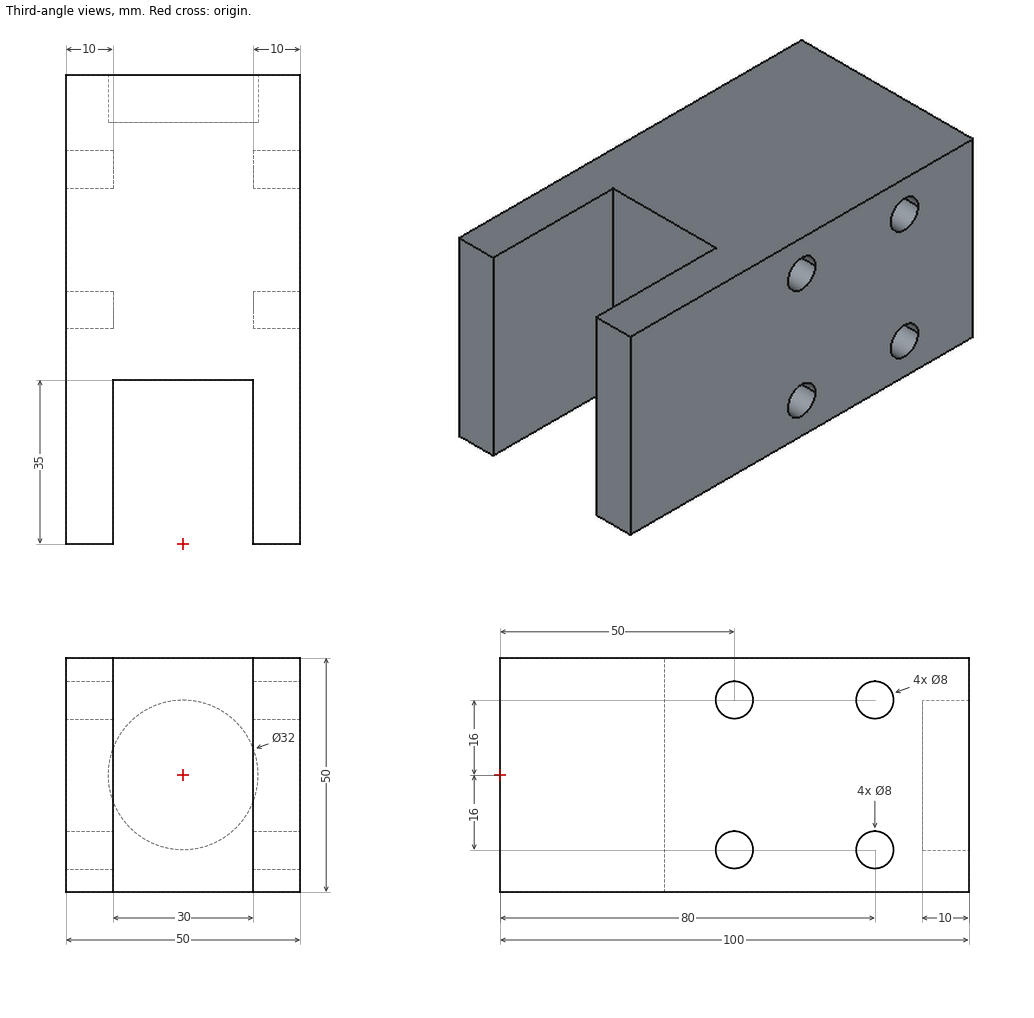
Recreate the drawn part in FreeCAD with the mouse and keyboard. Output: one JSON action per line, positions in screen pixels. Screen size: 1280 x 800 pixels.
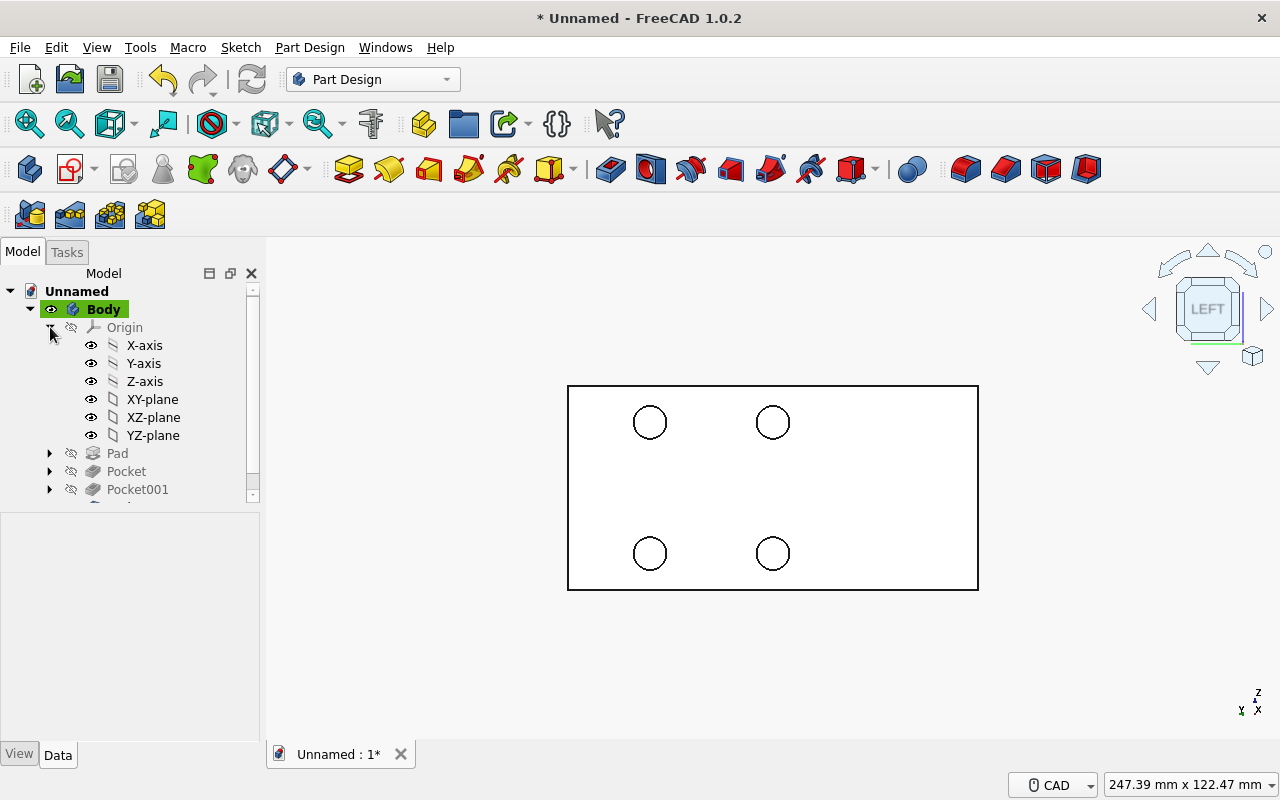
{"action": "left_click", "coordinate": [136, 435]}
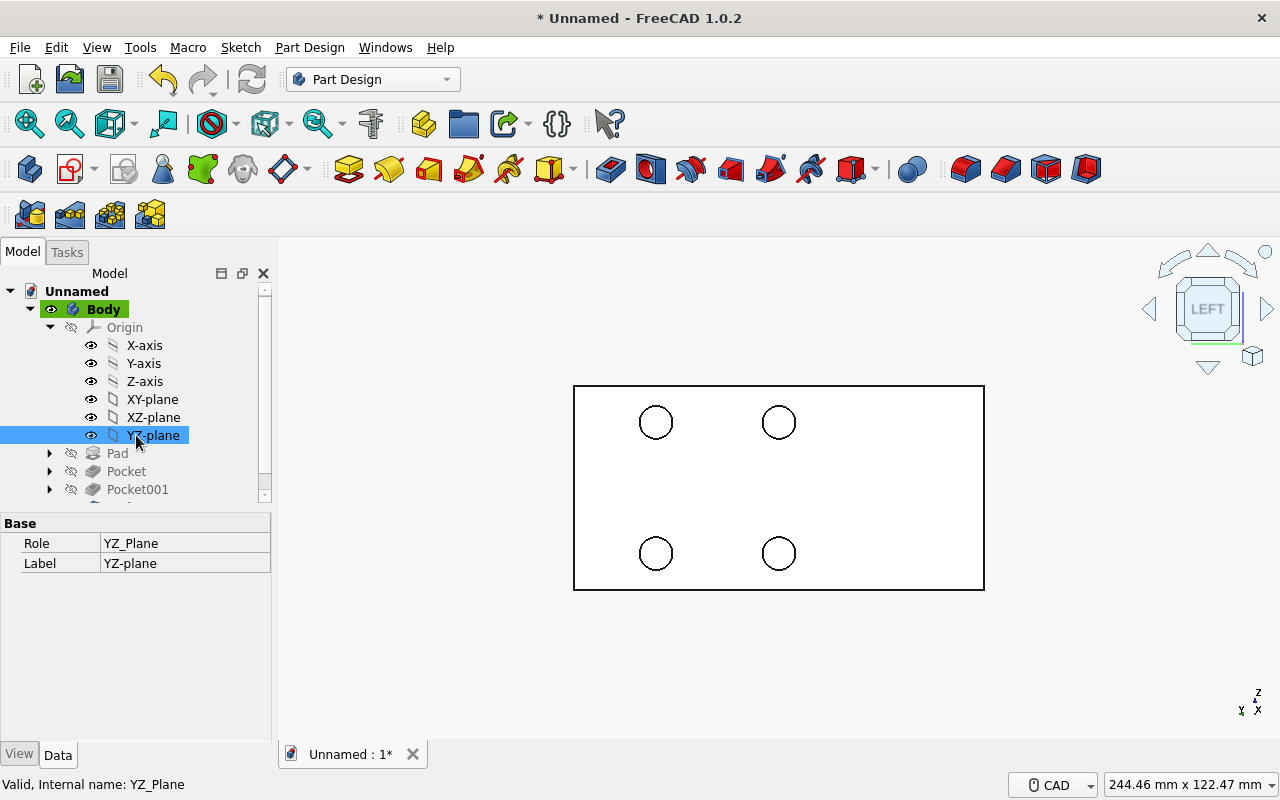
{"action": "left_click", "coordinate": [284, 170]}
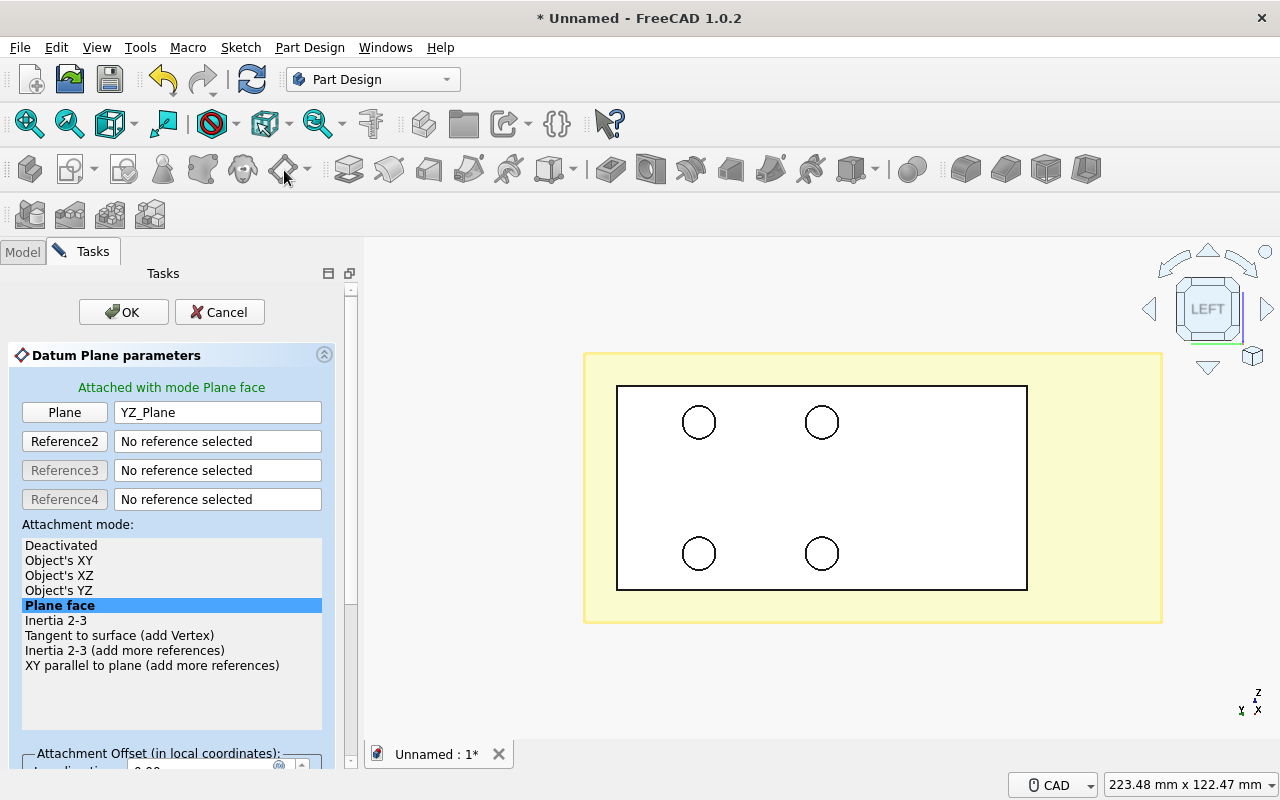
{"action": "scroll", "coordinate": [351, 526], "scroll_direction": "down", "scroll_amount": 3}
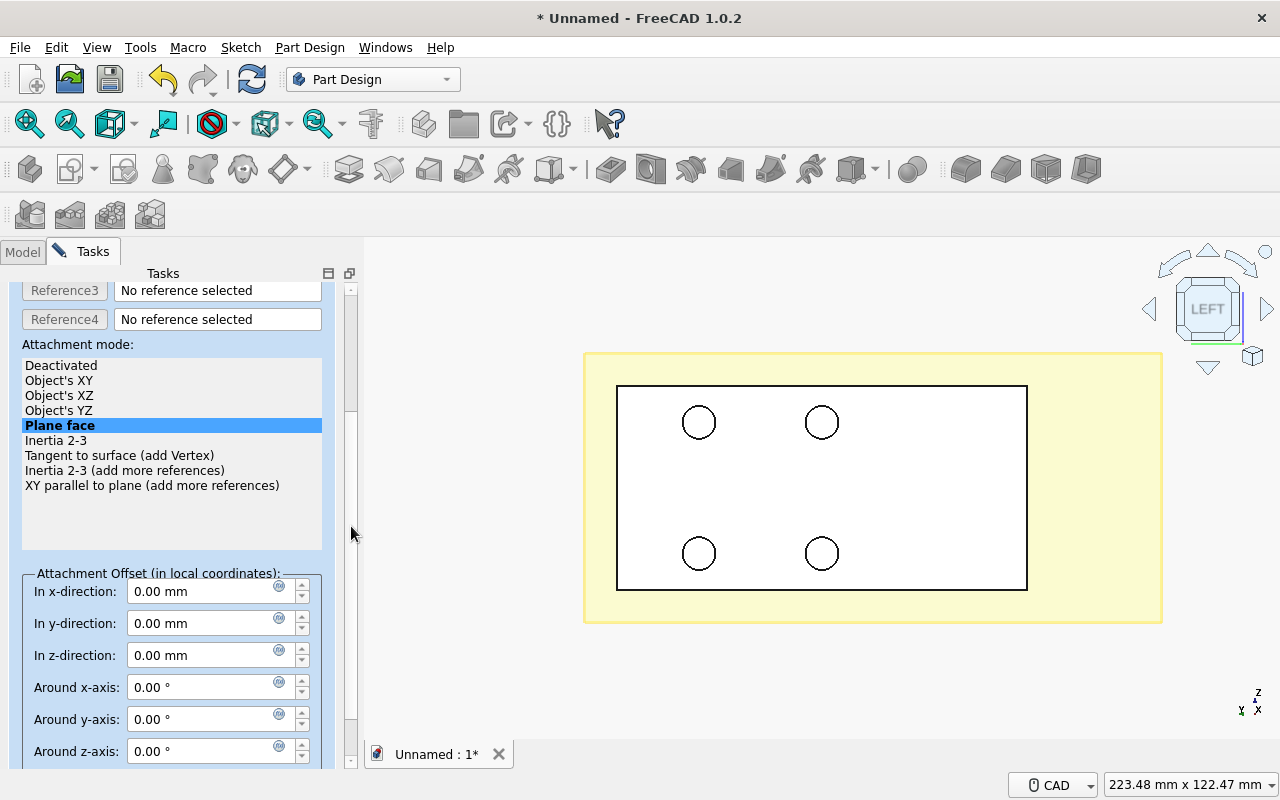
{"action": "triple_click", "coordinate": [210, 655]}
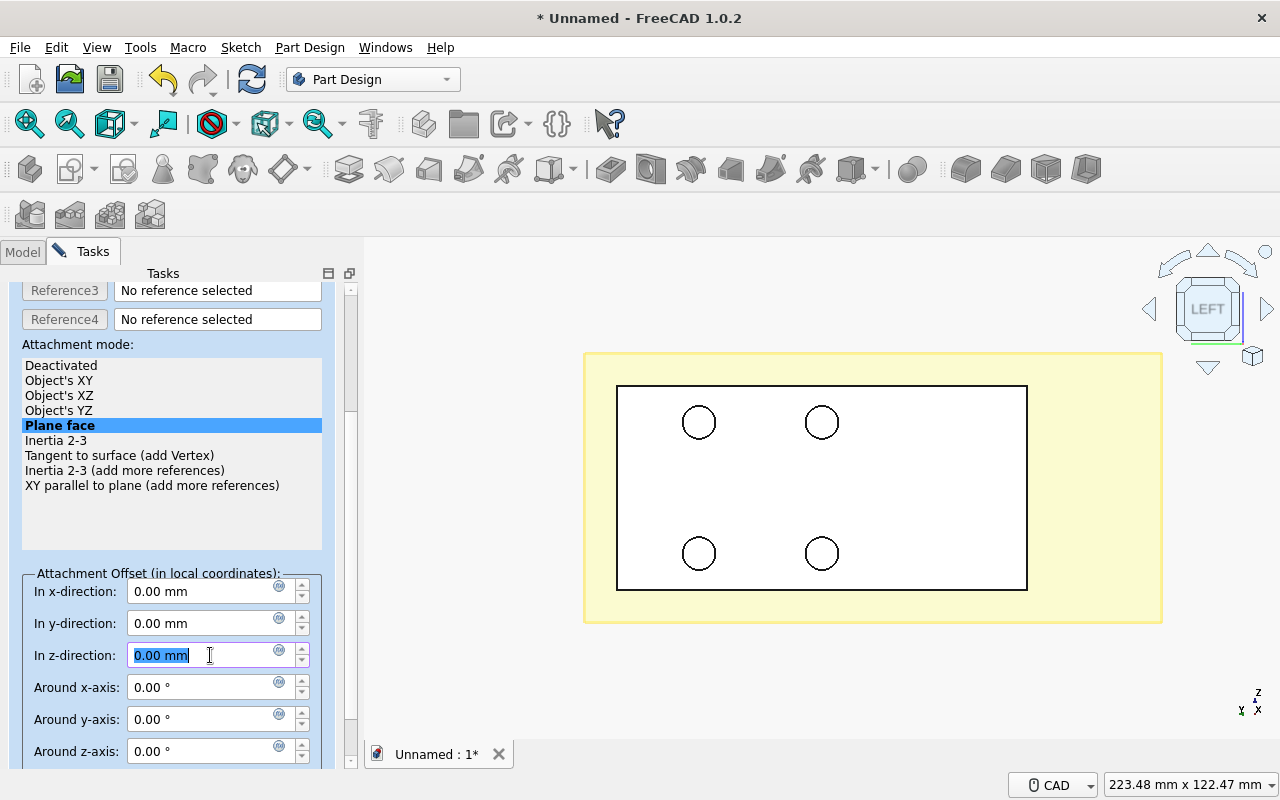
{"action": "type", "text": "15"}
{"action": "key", "text": "Tab"}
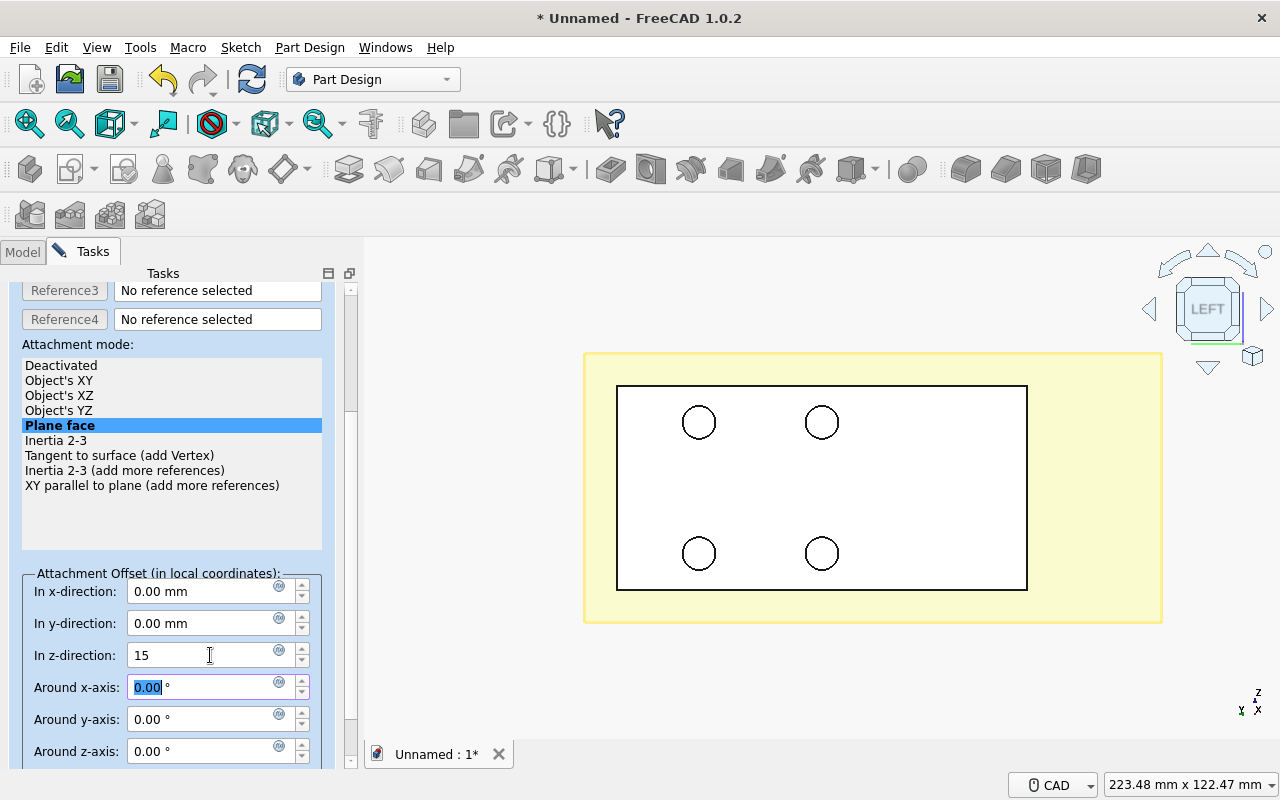
{"action": "scroll", "coordinate": [351, 526], "scroll_direction": "up", "scroll_amount": 4}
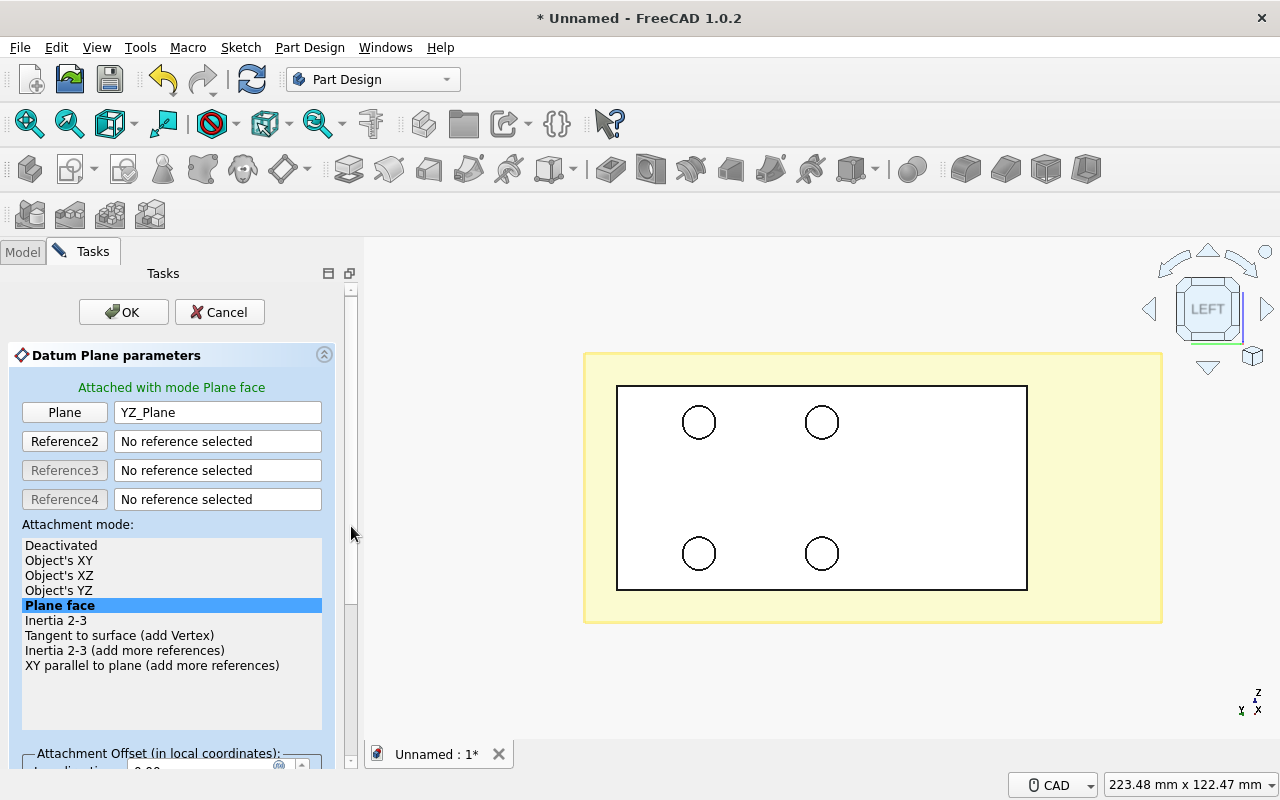
{"action": "left_click", "coordinate": [124, 312]}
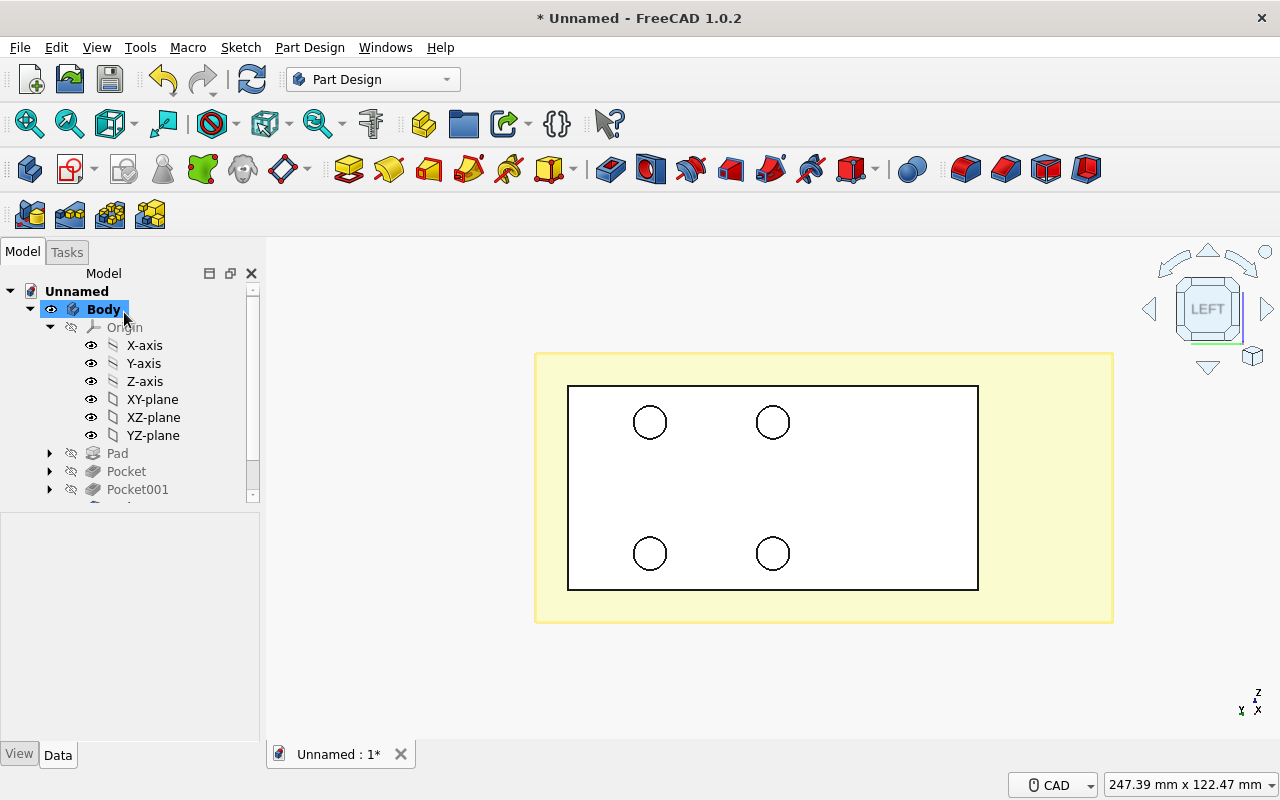
{"action": "scroll", "coordinate": [100, 395], "scroll_direction": "down", "scroll_amount": 3}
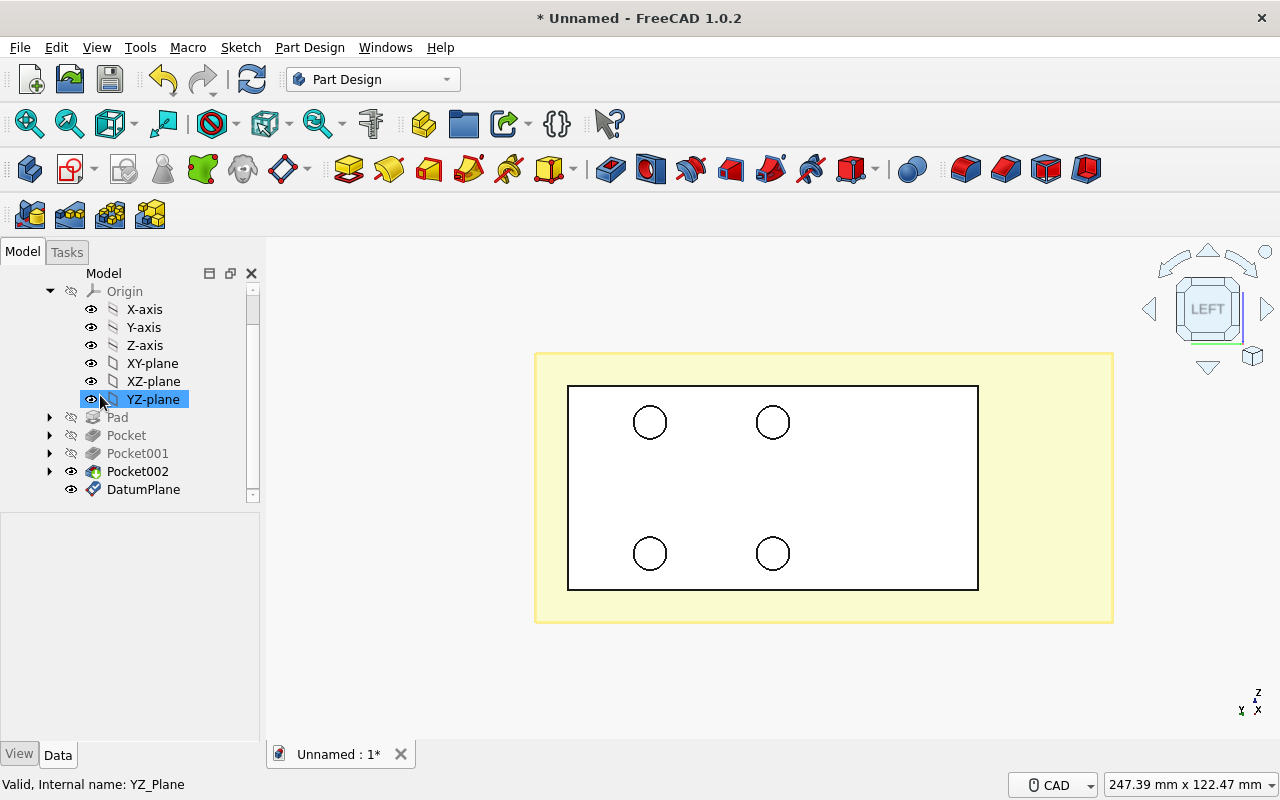
{"action": "left_click", "coordinate": [116, 489]}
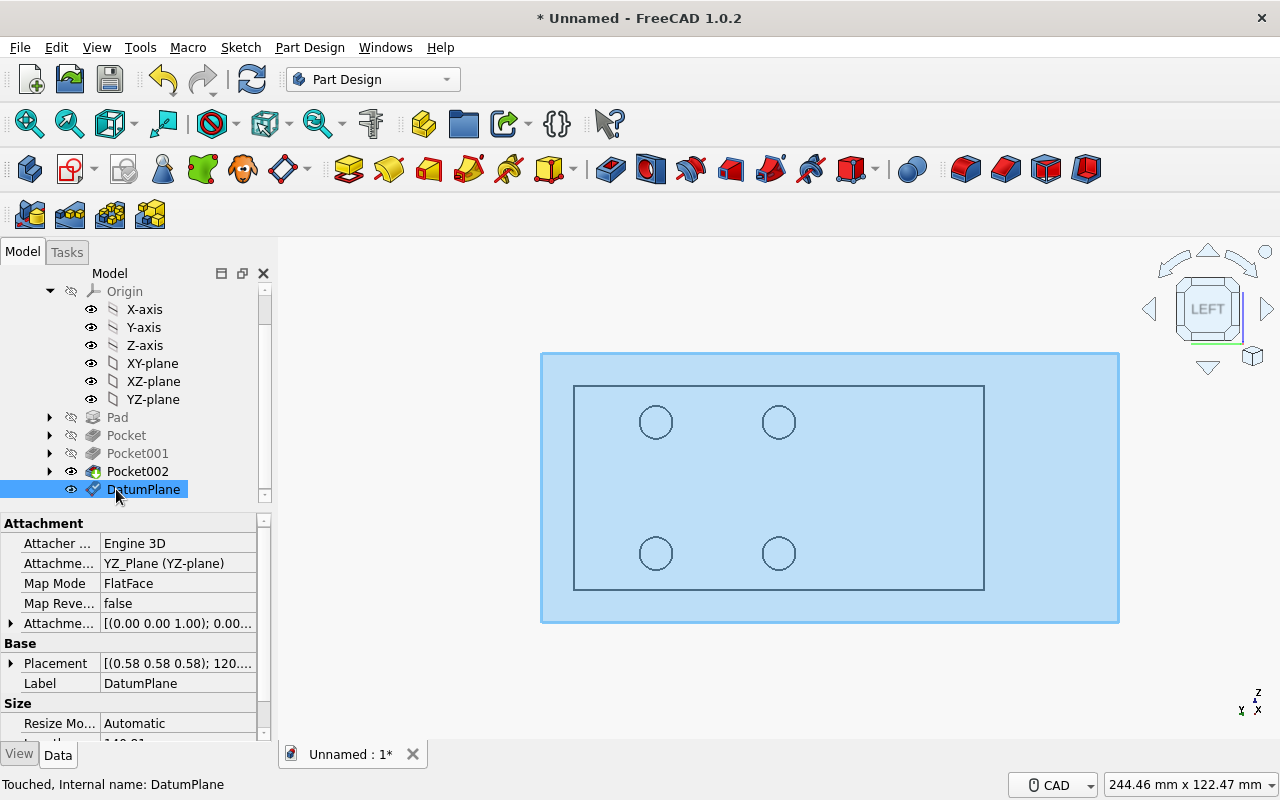
{"action": "left_click", "coordinate": [70, 170]}